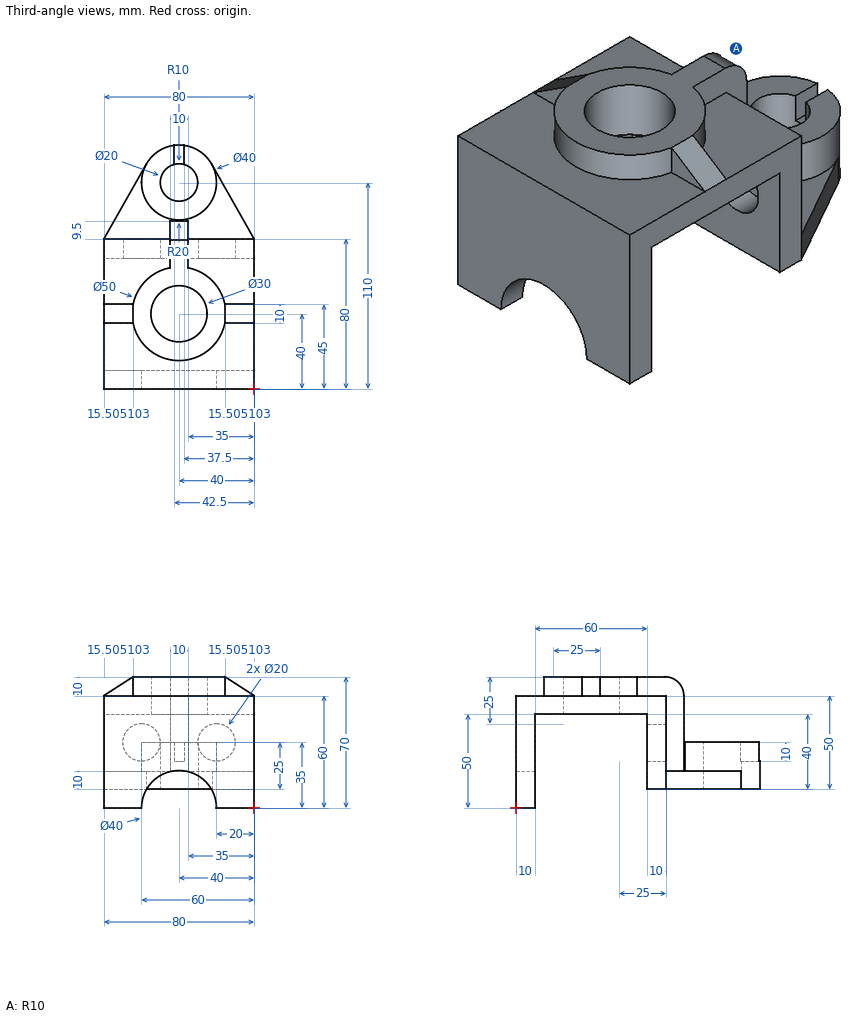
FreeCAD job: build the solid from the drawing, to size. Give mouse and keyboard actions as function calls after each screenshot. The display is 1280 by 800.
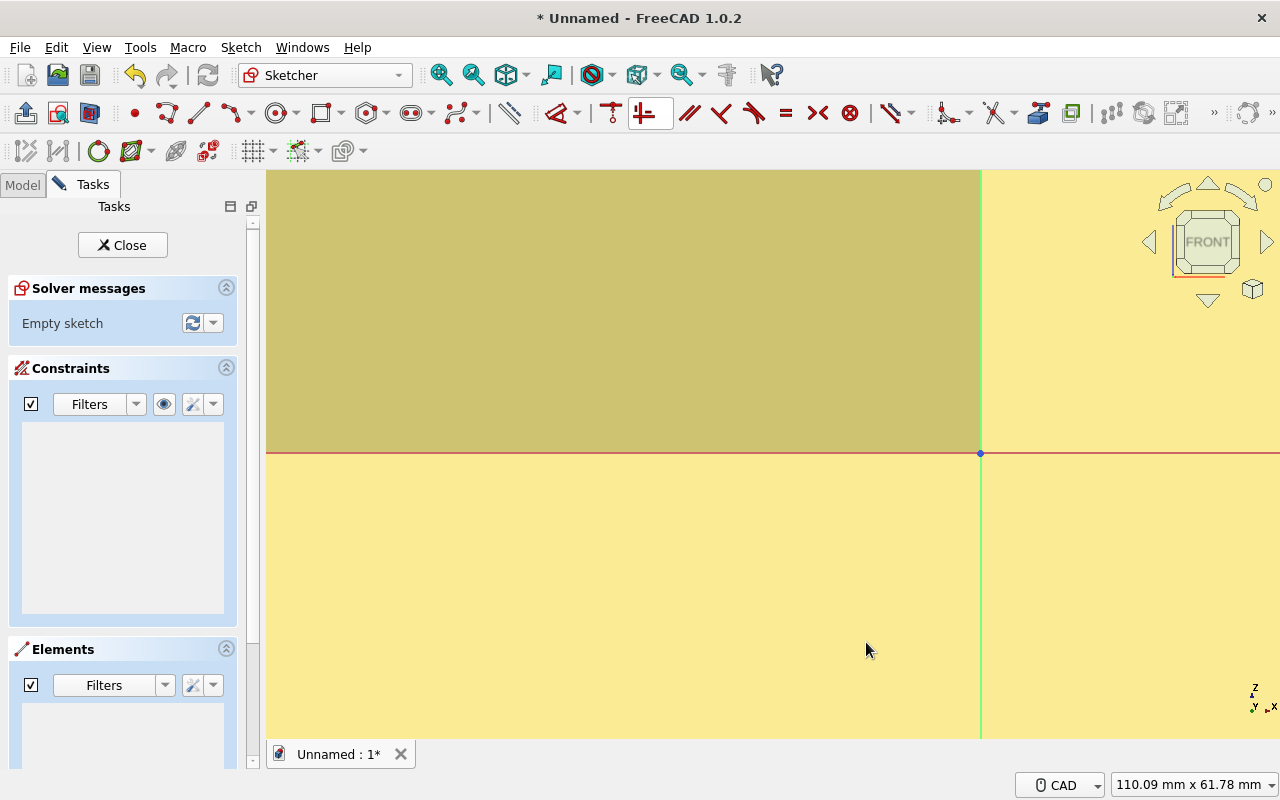
click(276, 114)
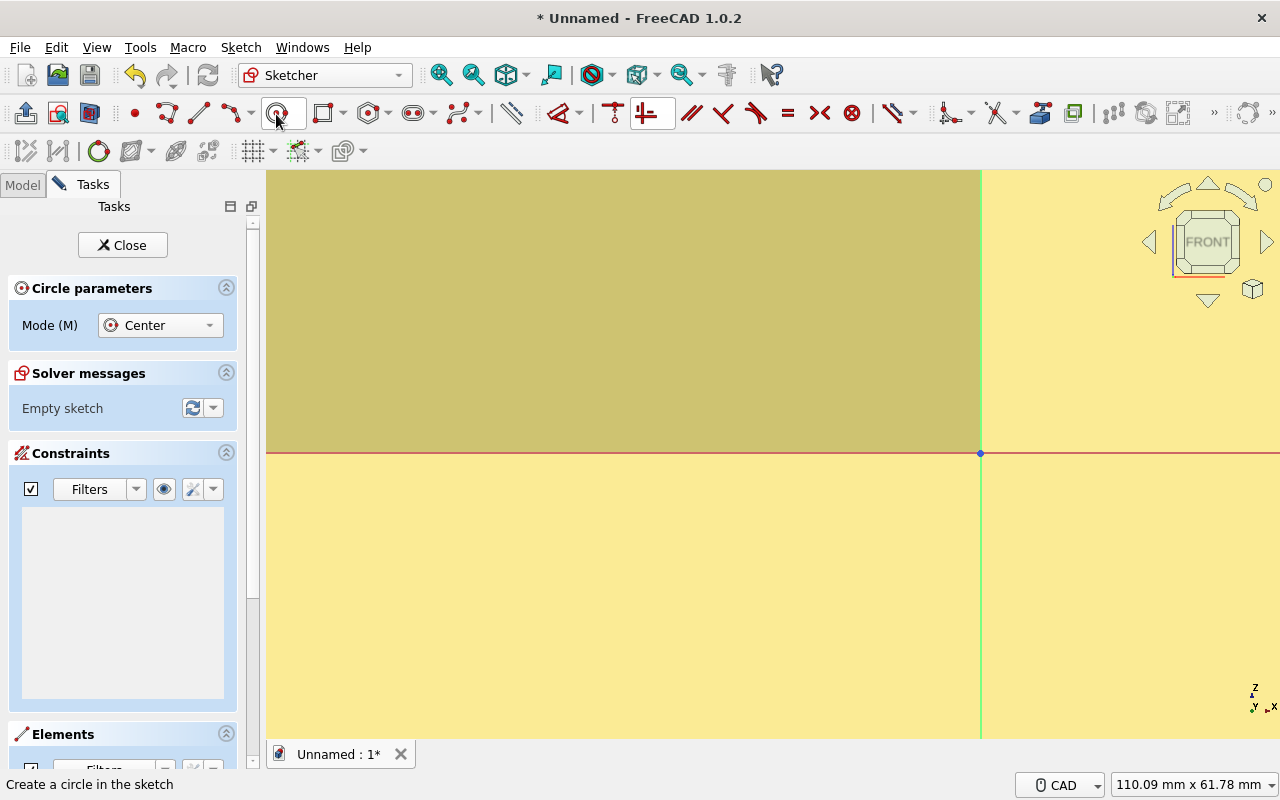
click(612, 453)
move(742, 323)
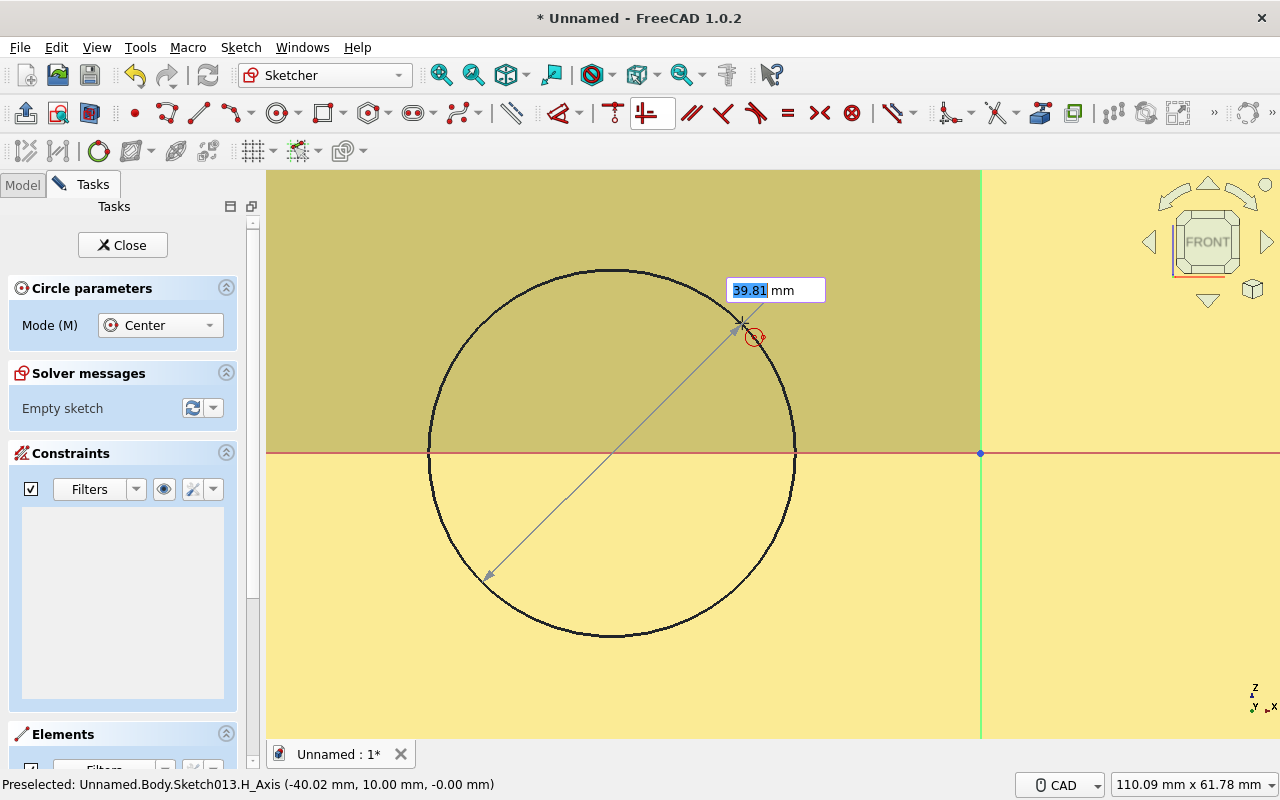
text(40)
key(Return)
key(Escape)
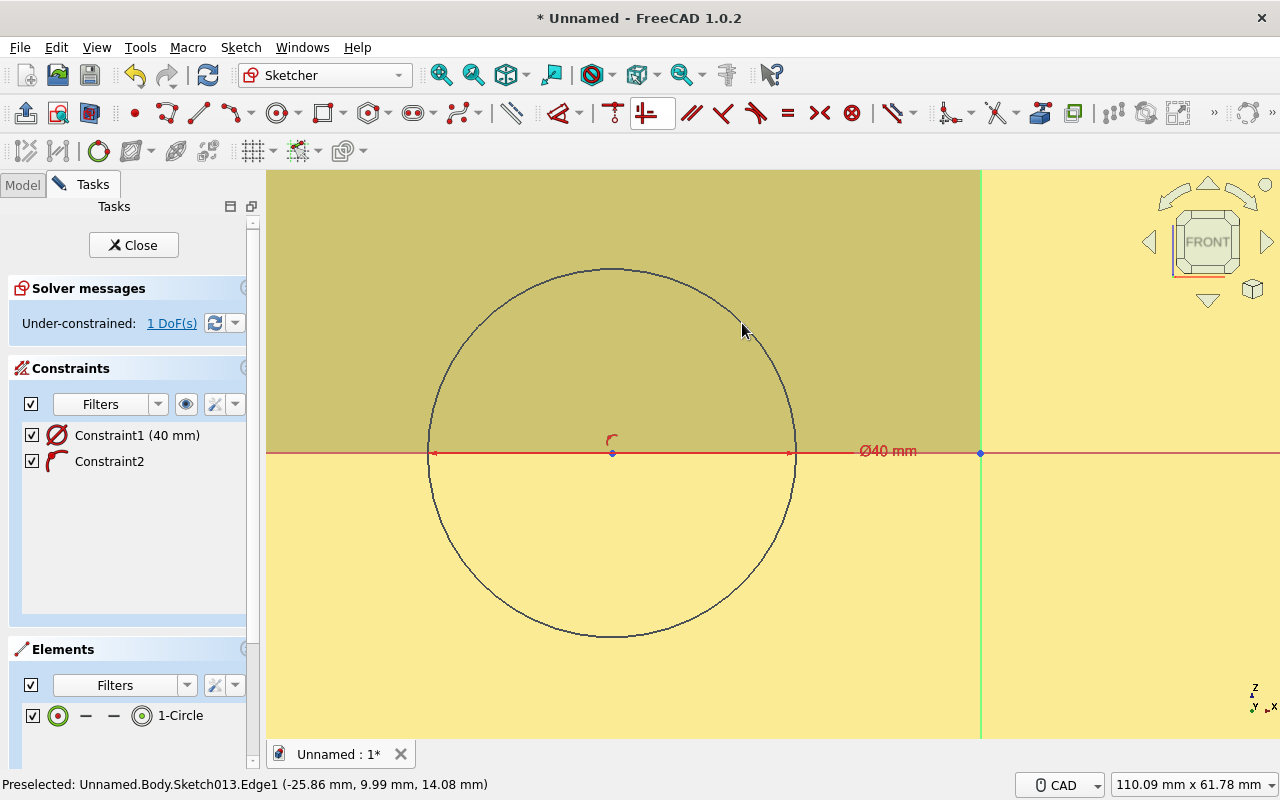
click(558, 114)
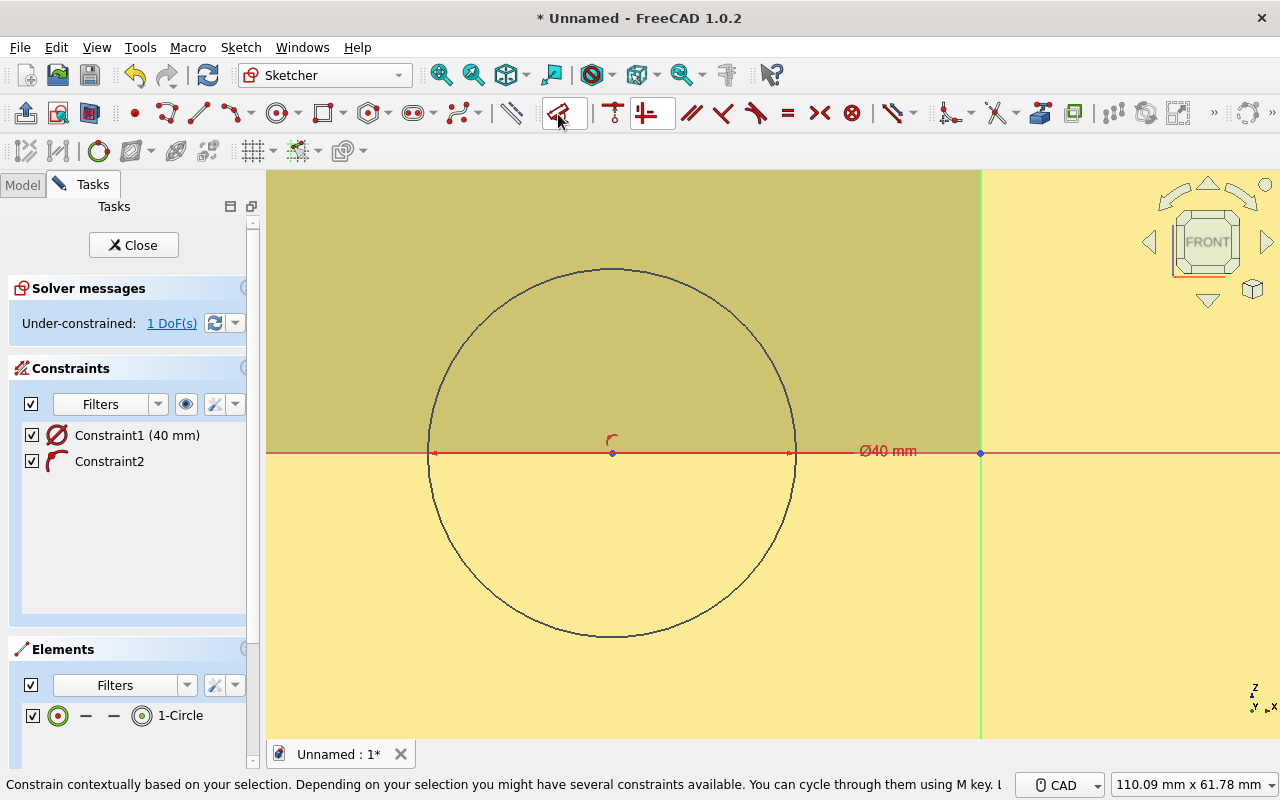
click(612, 453)
click(712, 487)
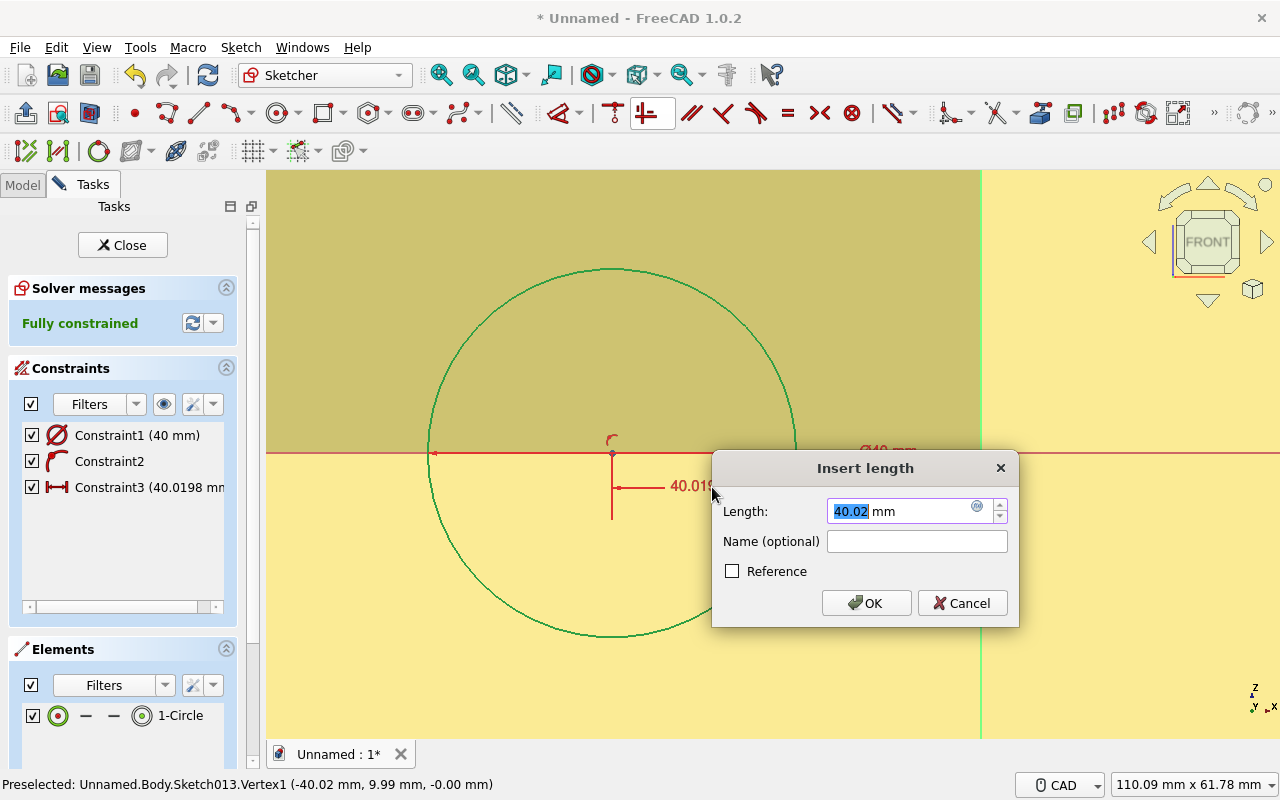
text(40)
key(Return)
key(Escape)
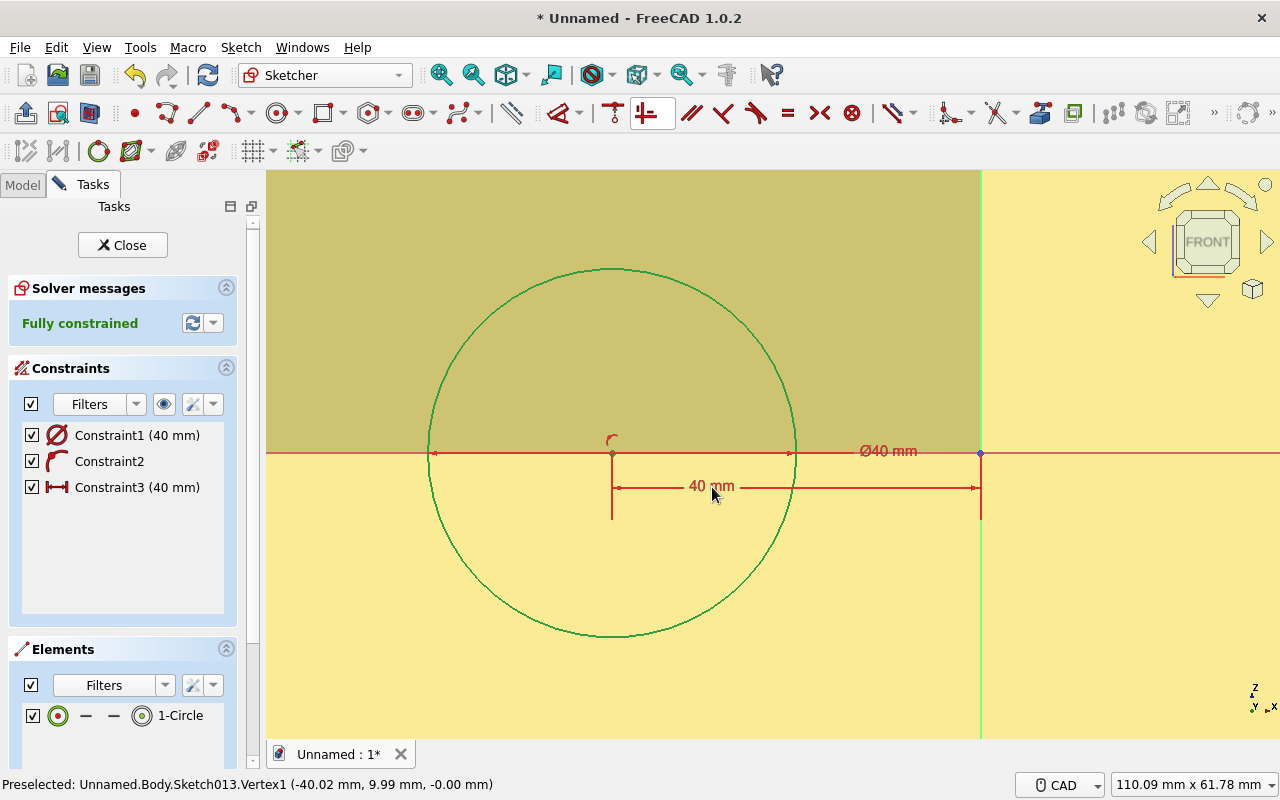
click(123, 245)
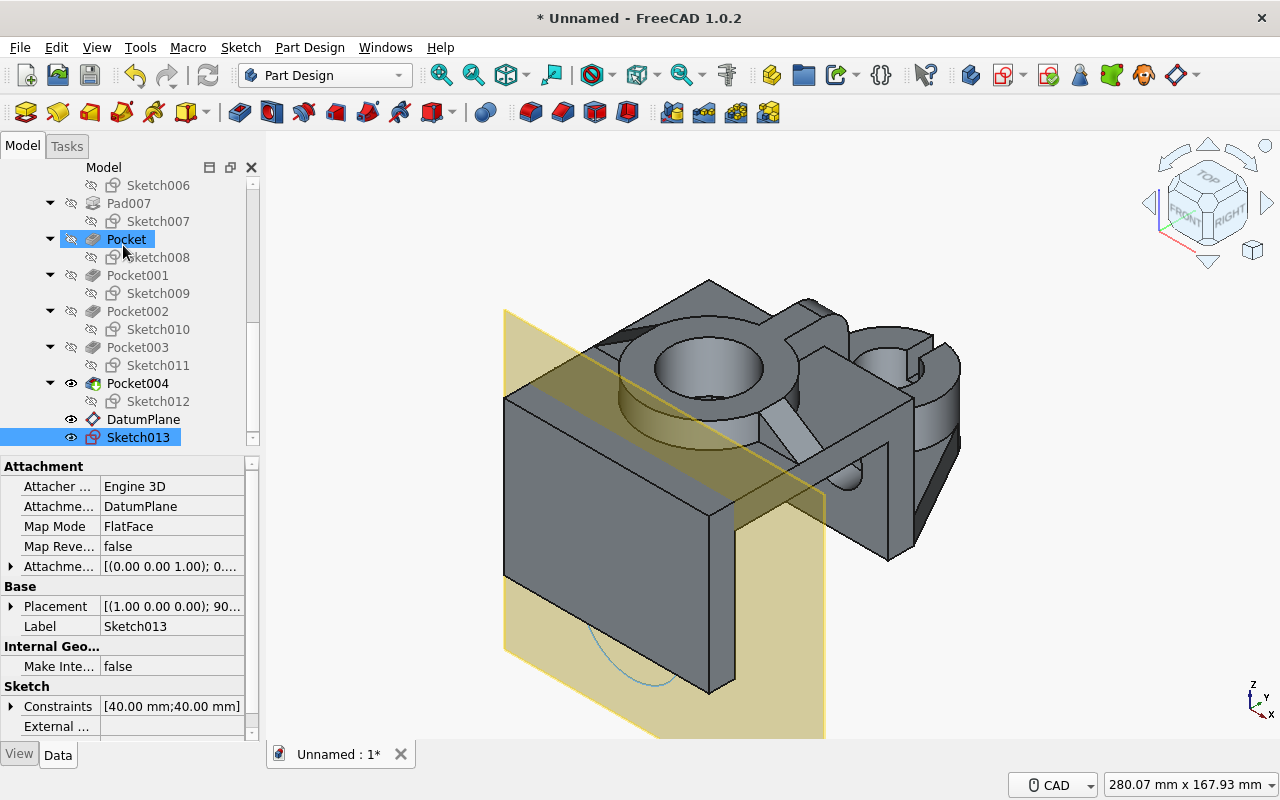
click(240, 112)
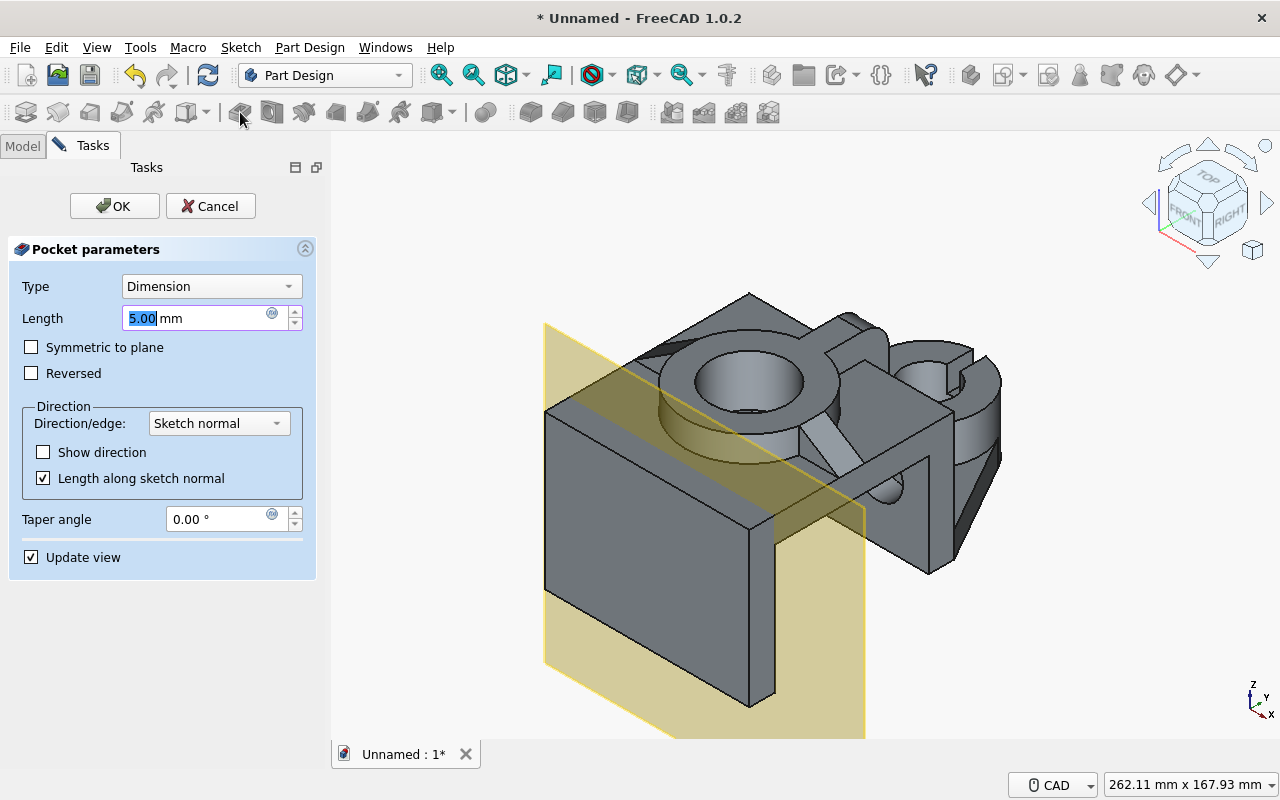
text(10)
key(Tab)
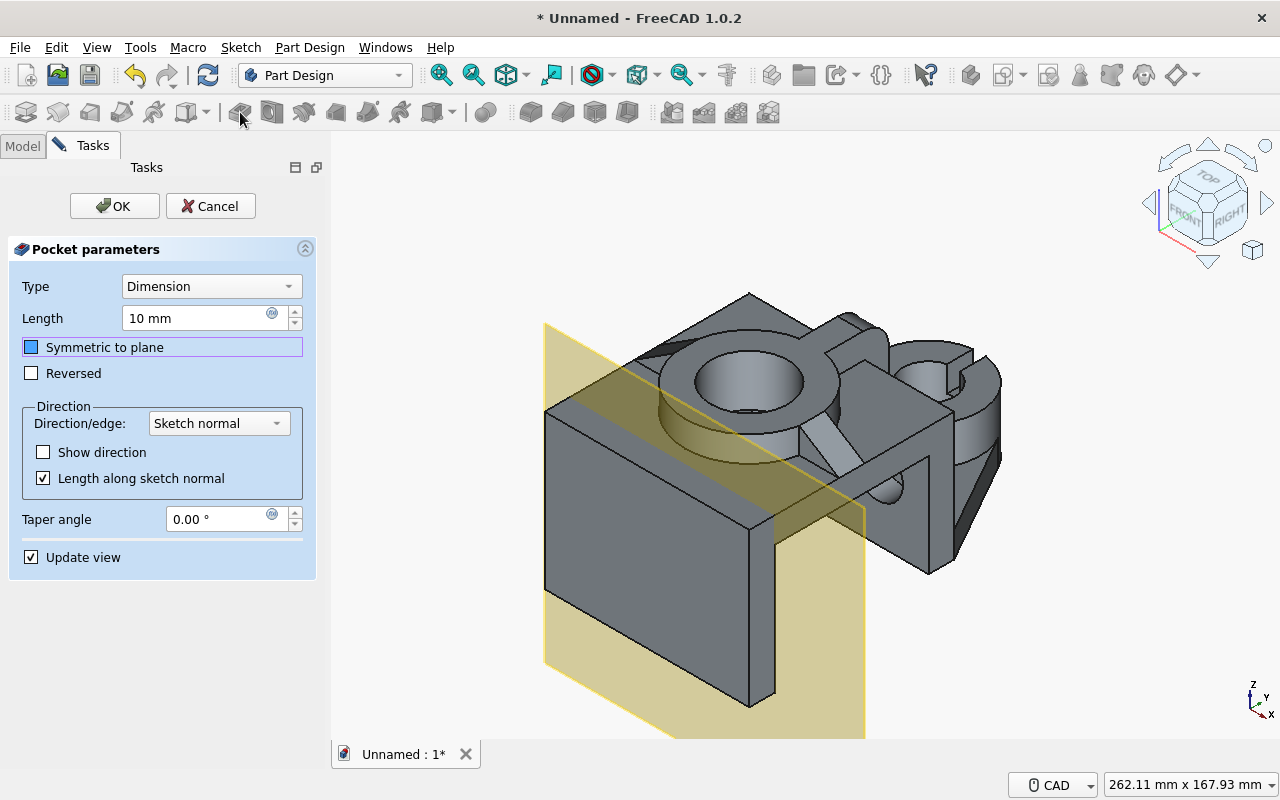
click(30, 373)